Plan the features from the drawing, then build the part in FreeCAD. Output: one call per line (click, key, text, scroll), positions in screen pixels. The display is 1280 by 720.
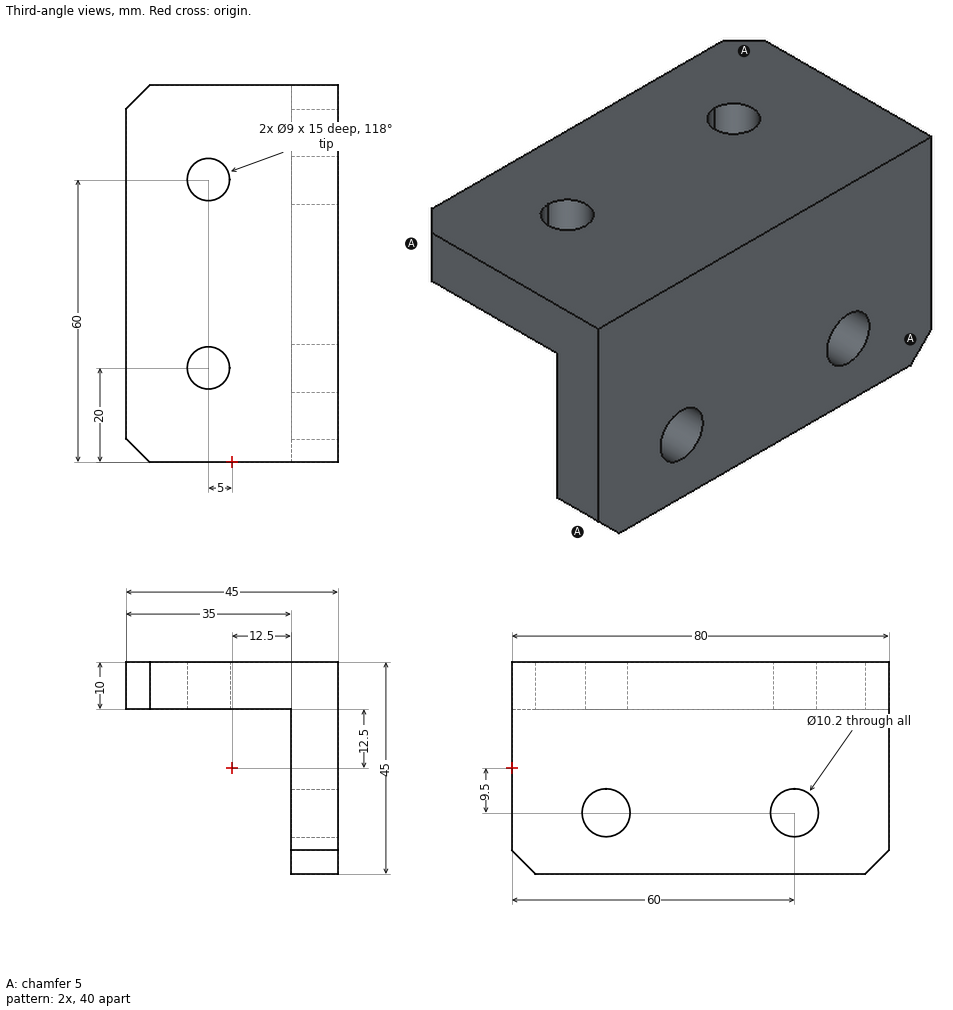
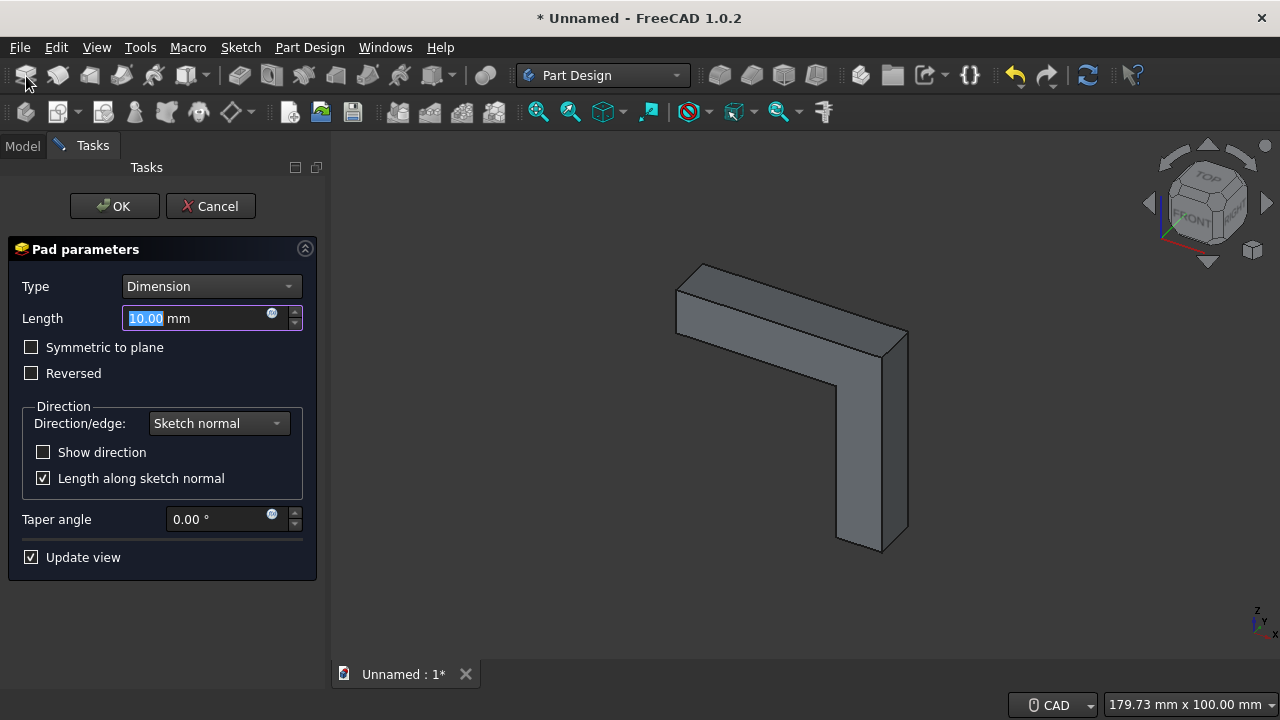
text(80)
key(Tab)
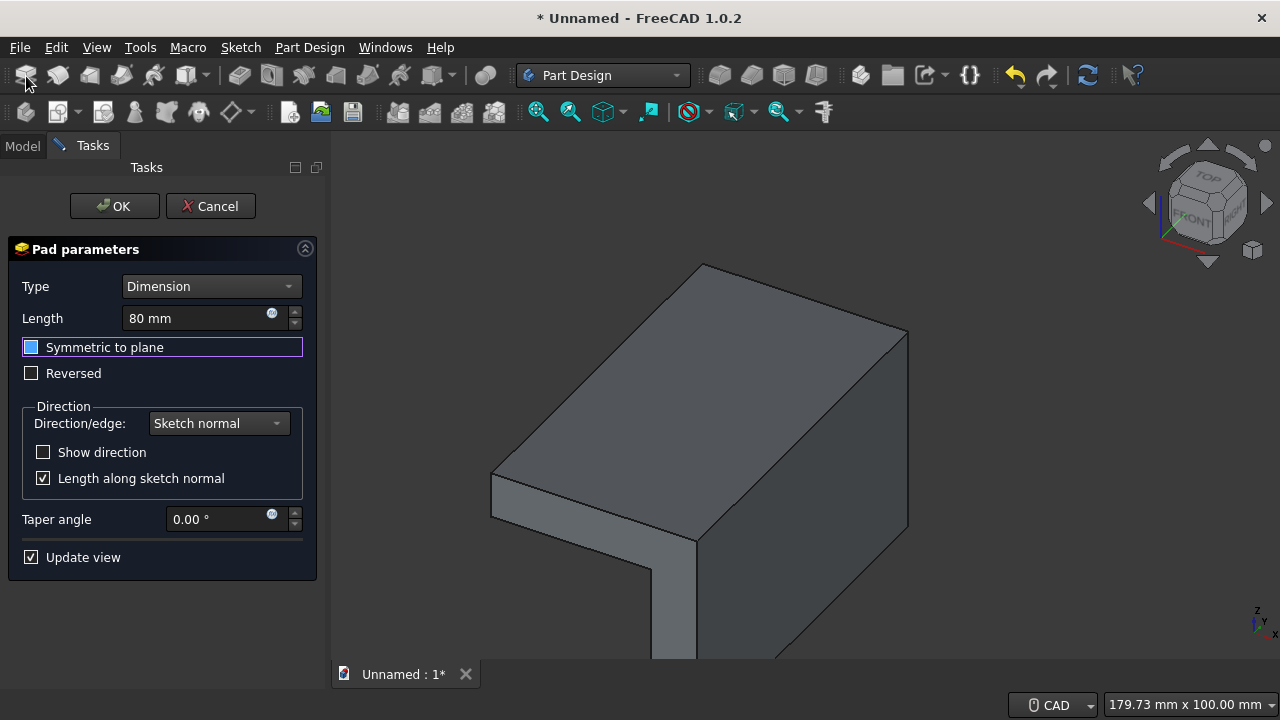
click(30, 373)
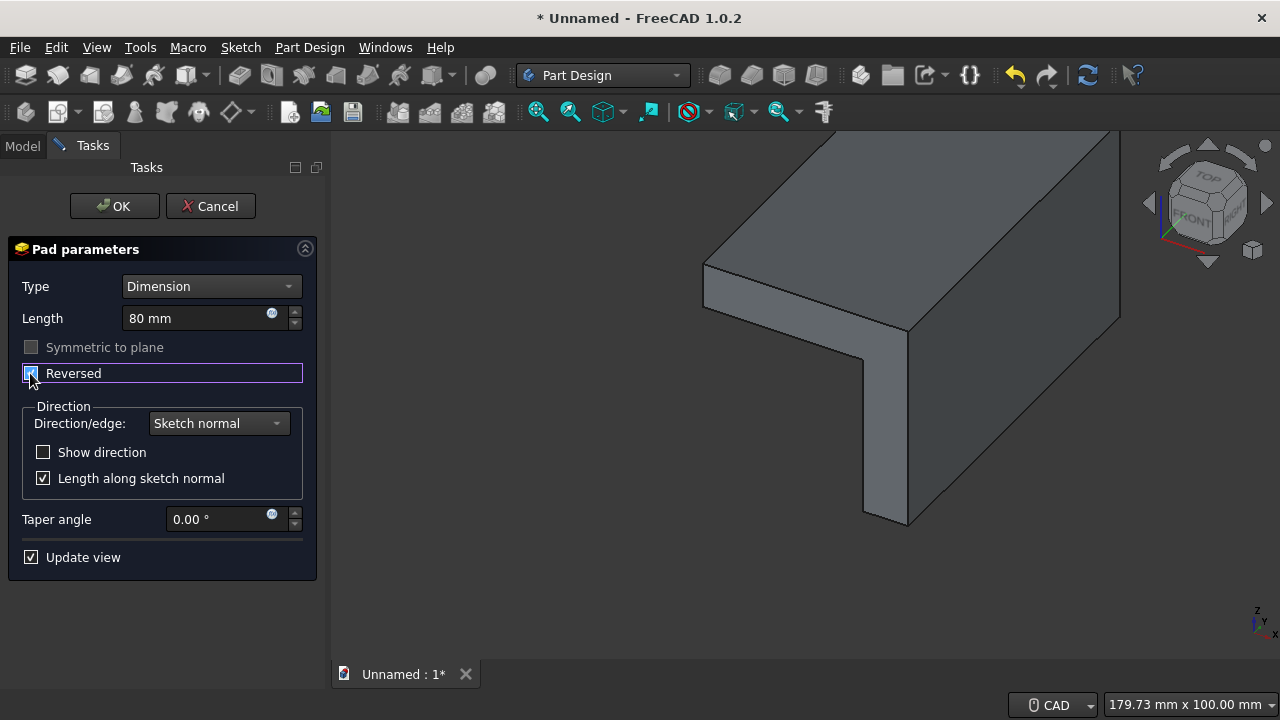
click(115, 206)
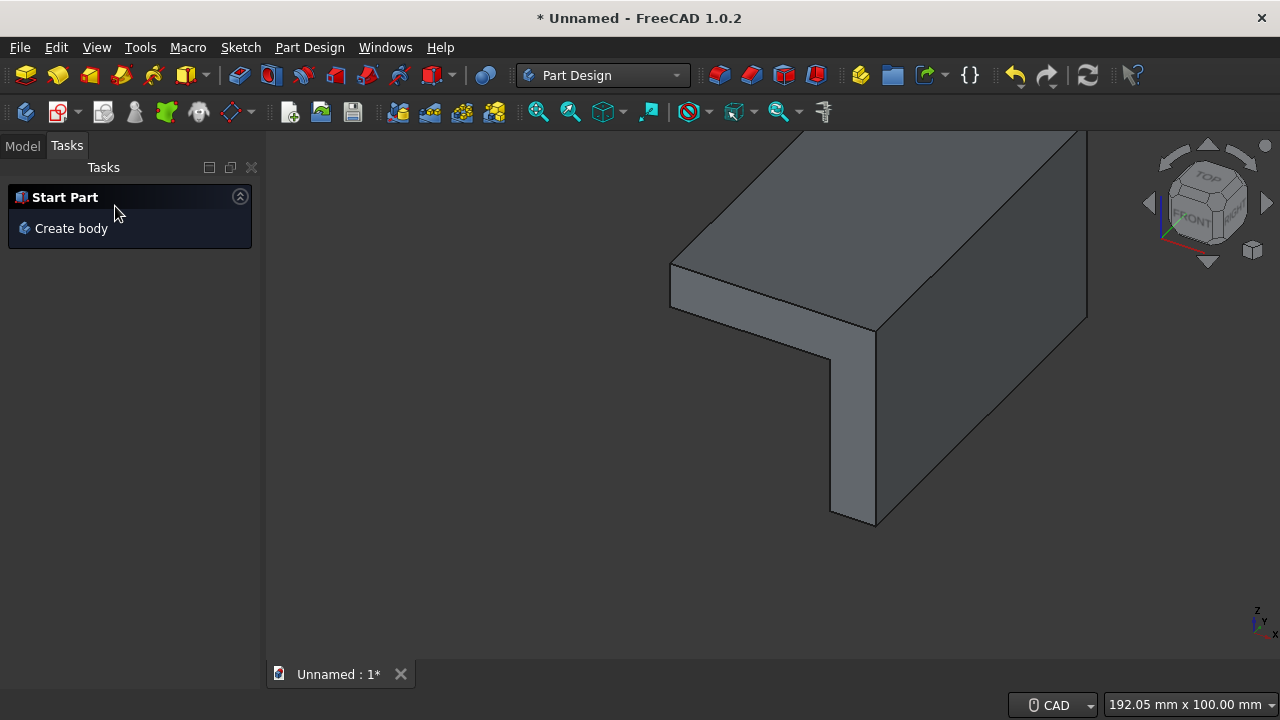
key(v)
key(f)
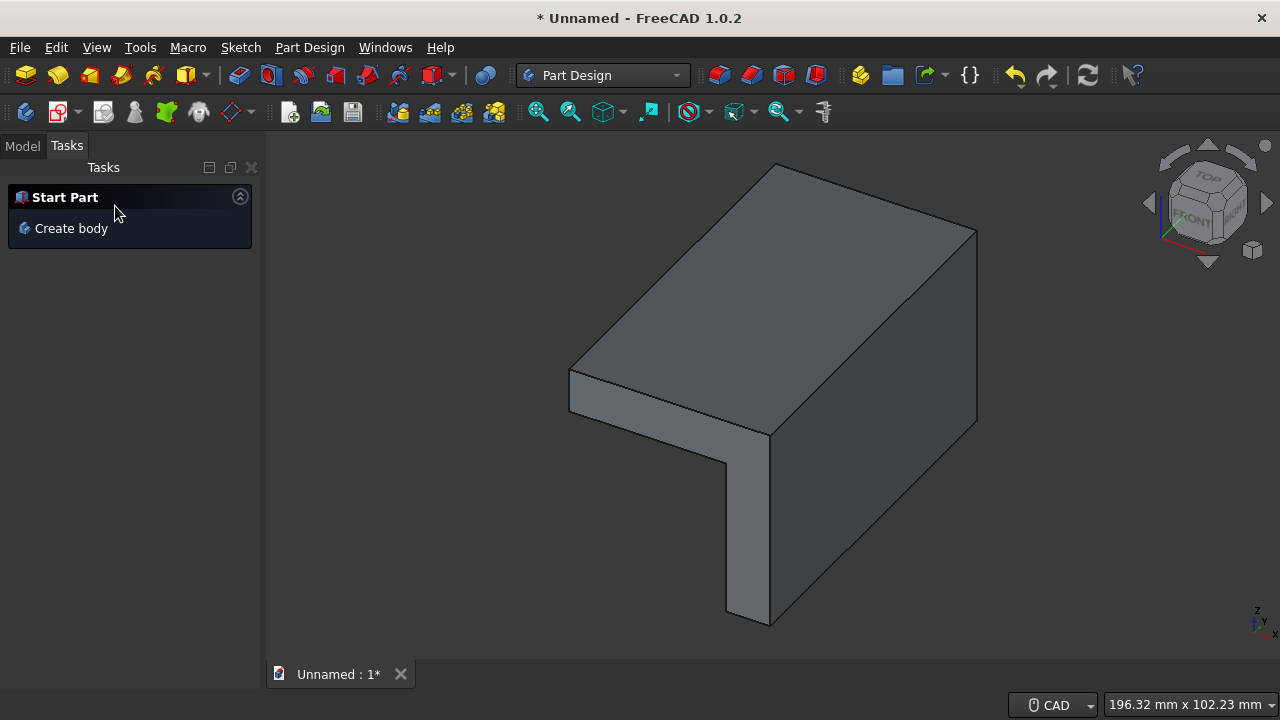
key(0)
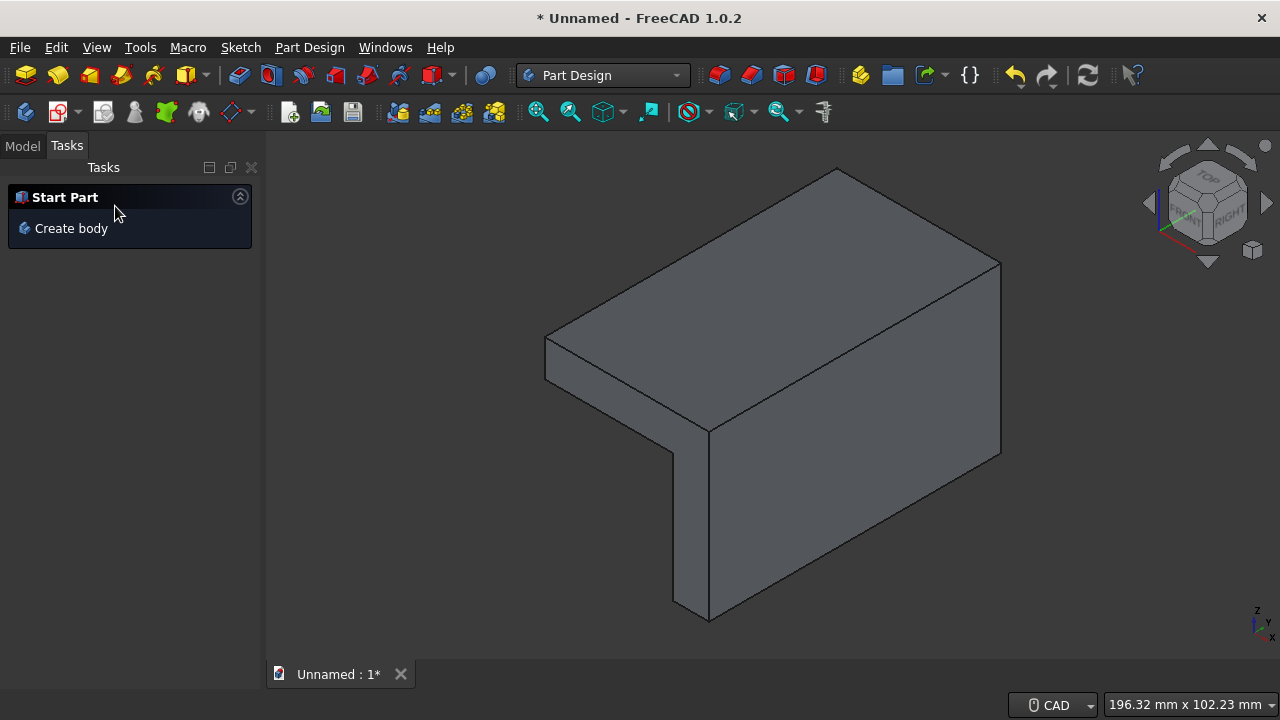
key(2)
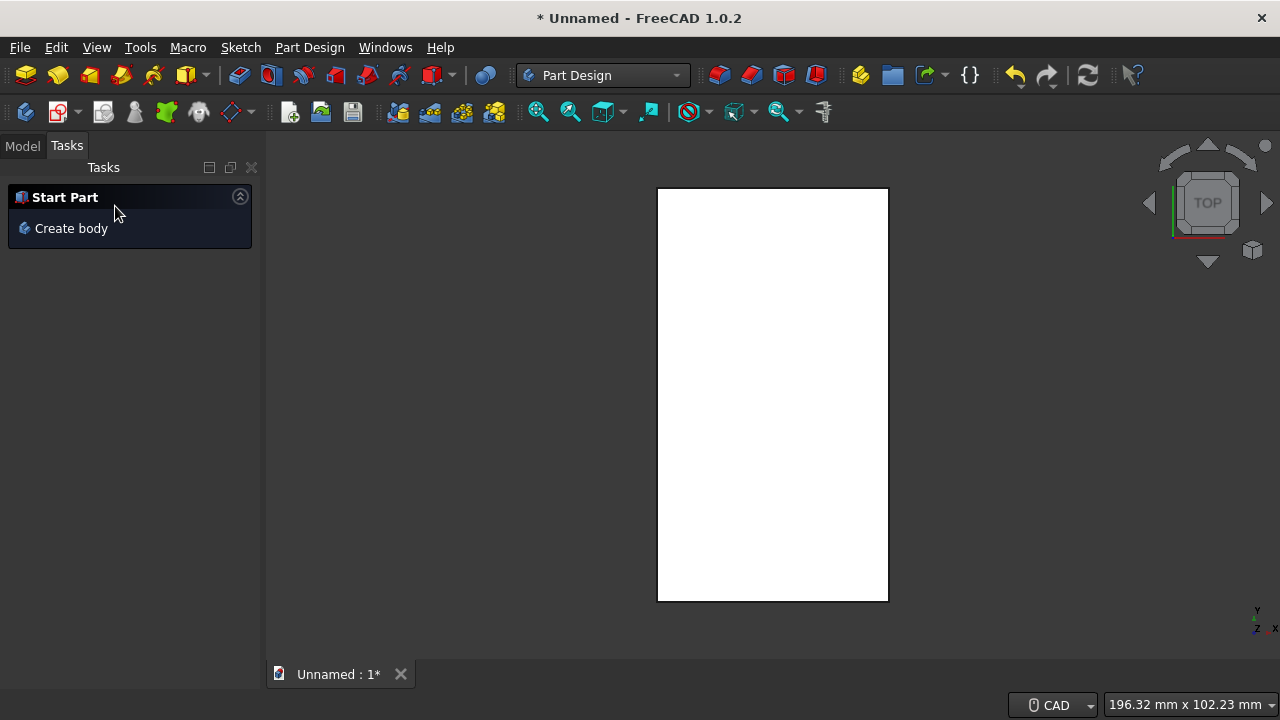
key(1)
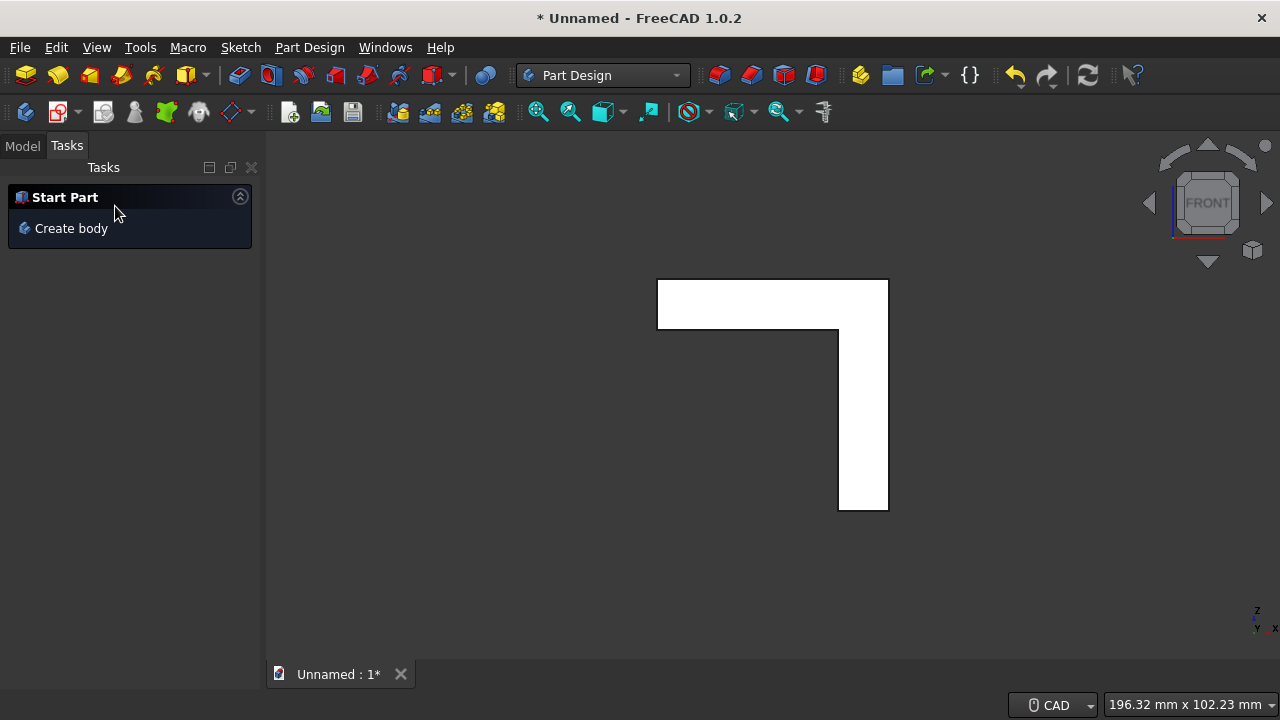
click(540, 112)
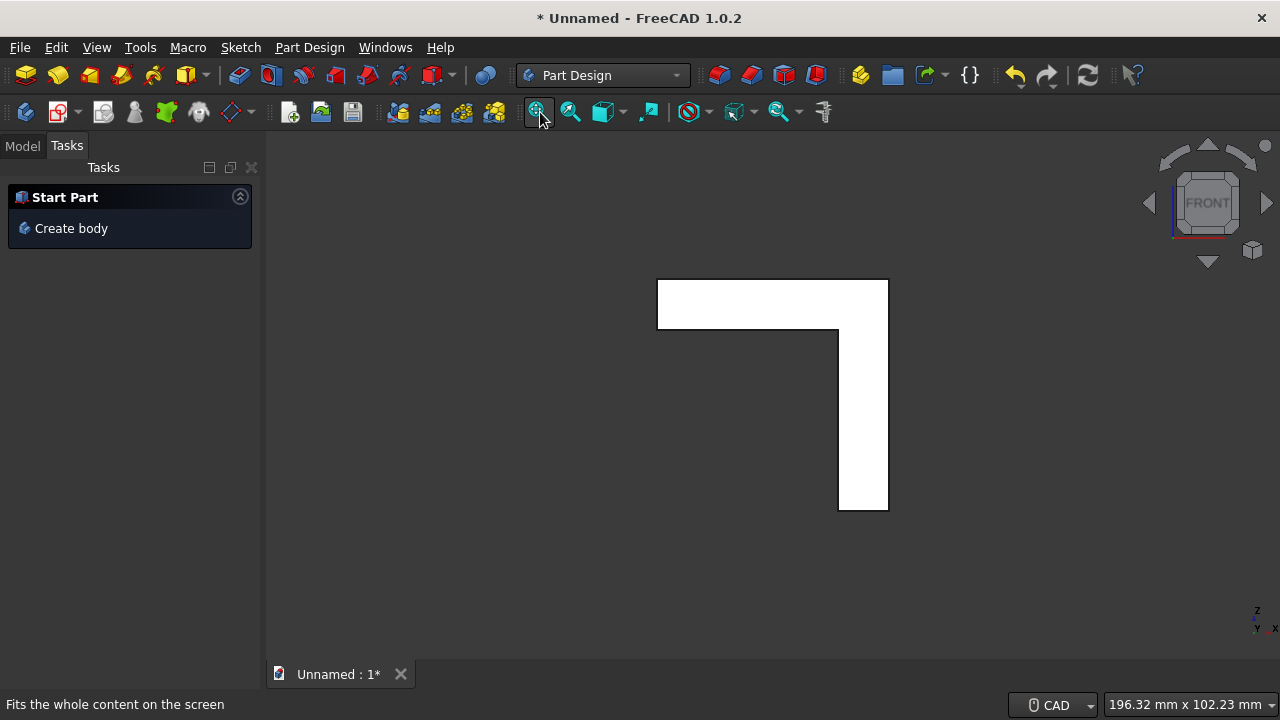
click(657, 309)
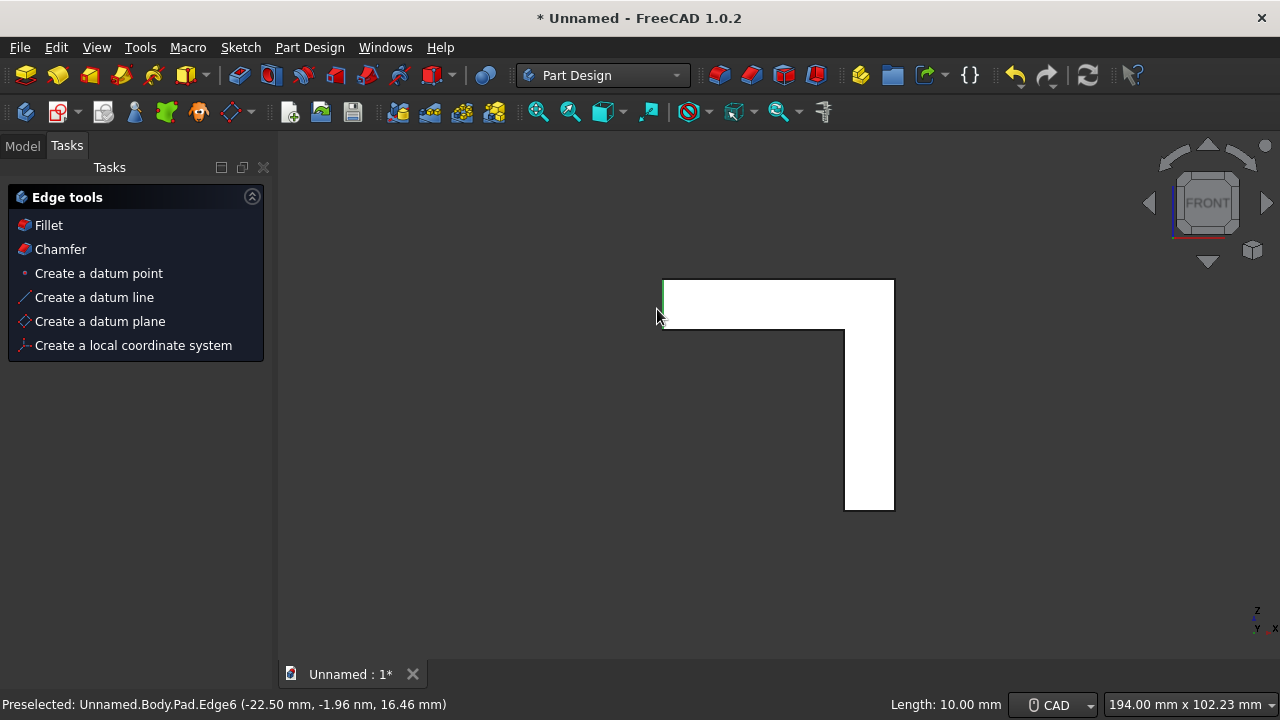
key(3)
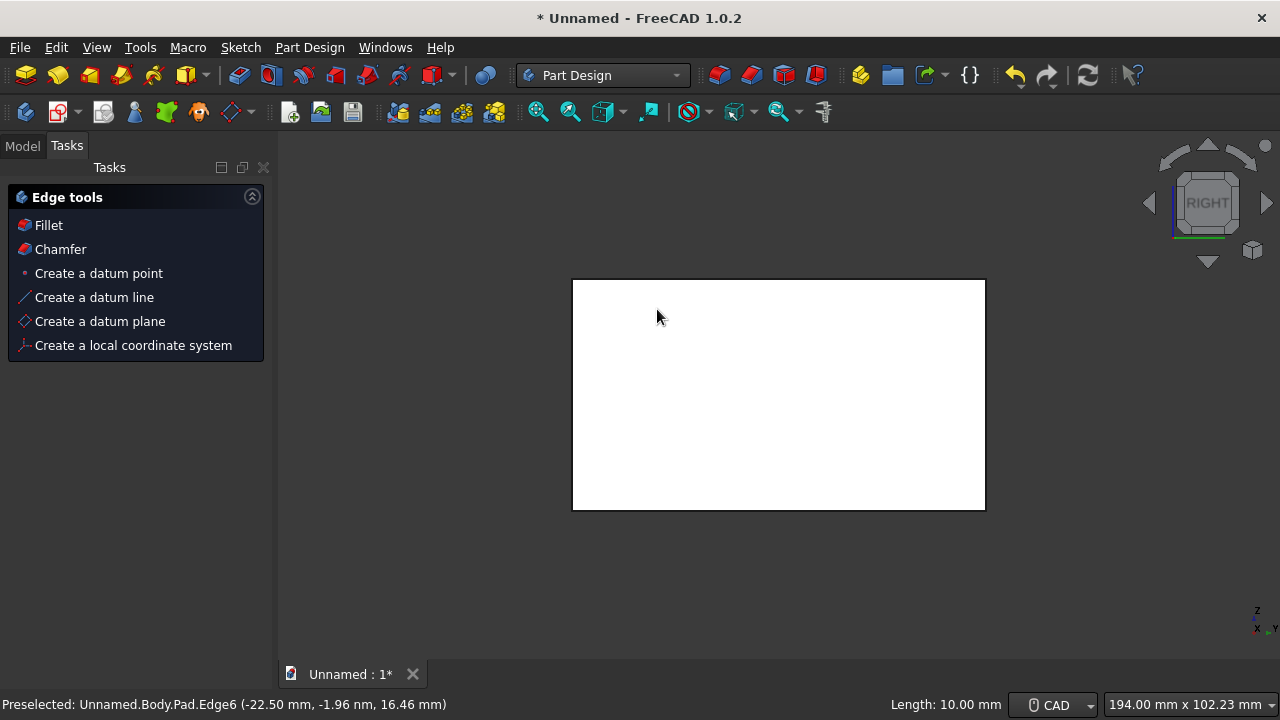
click(540, 112)